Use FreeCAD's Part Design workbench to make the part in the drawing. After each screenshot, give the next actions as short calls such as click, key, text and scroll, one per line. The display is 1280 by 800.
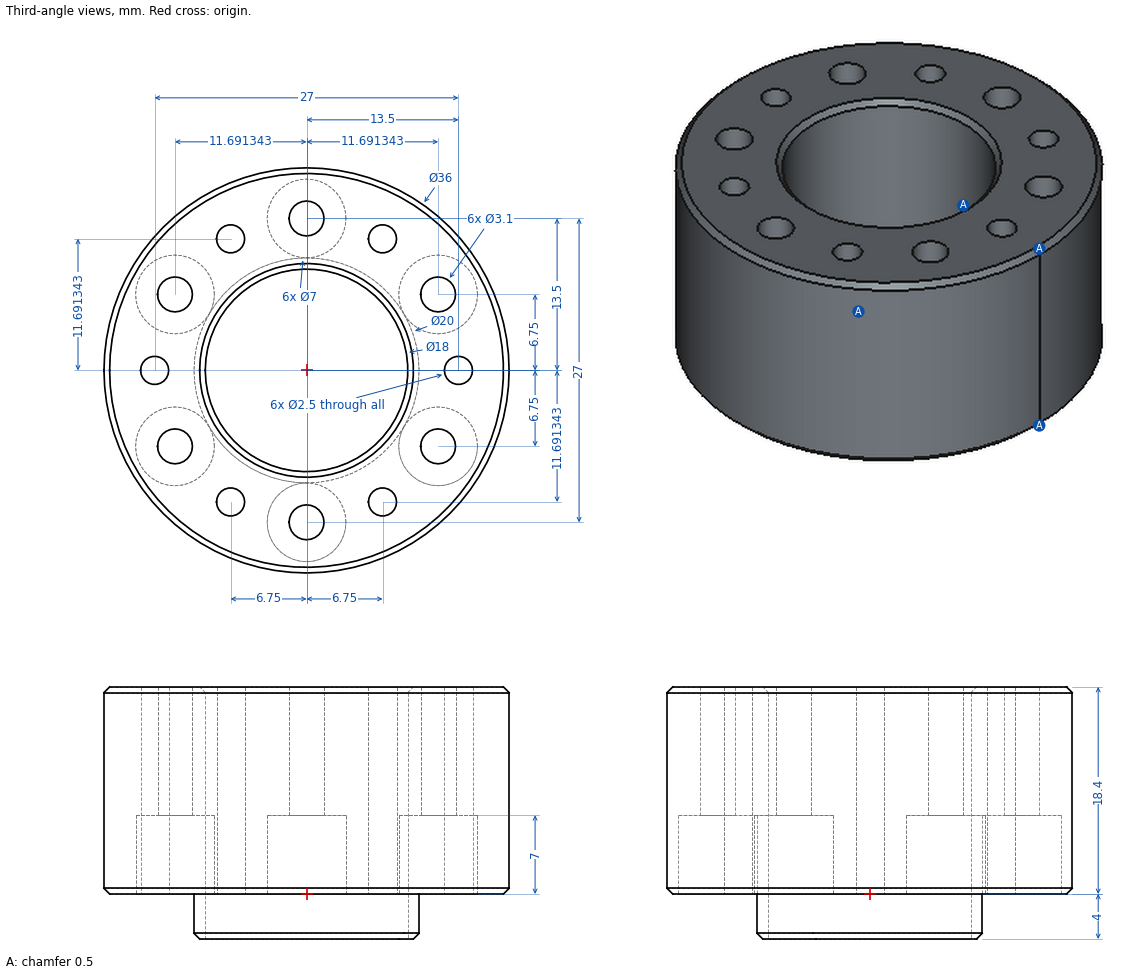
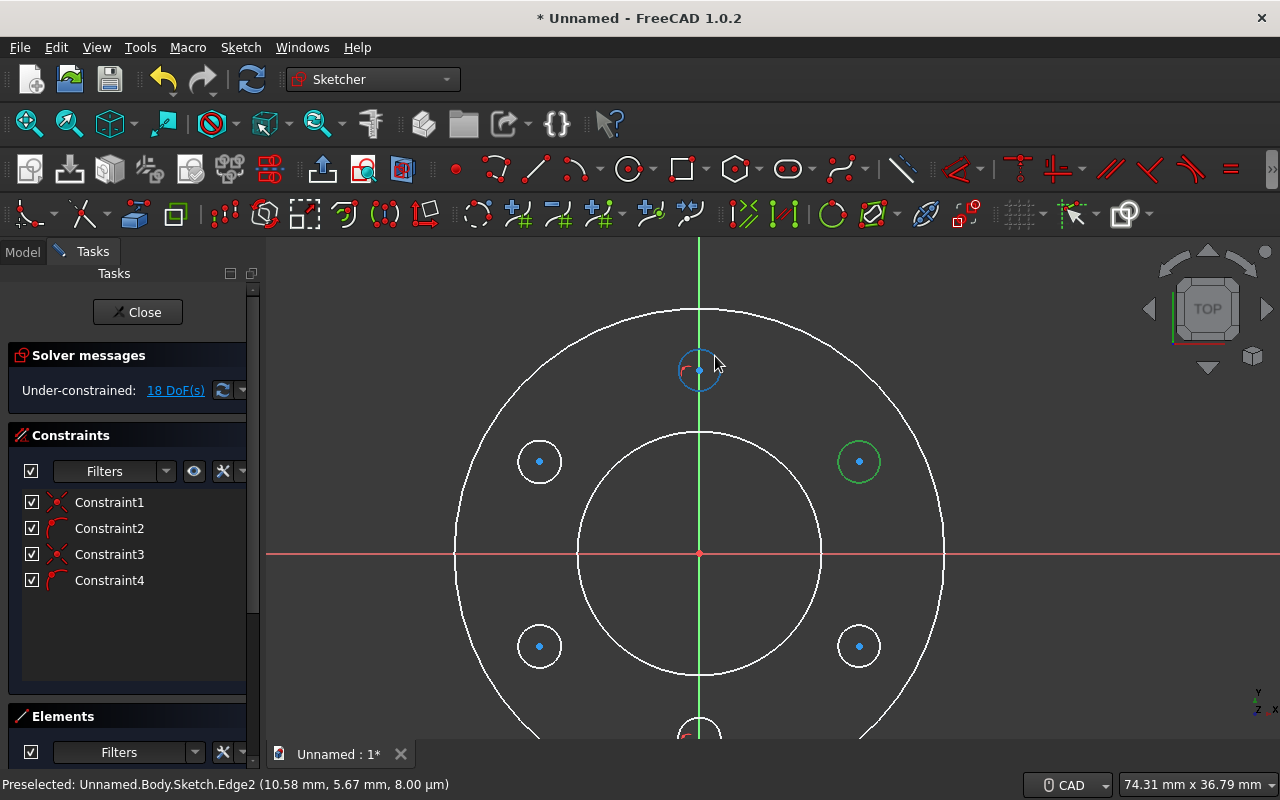
click(714, 355)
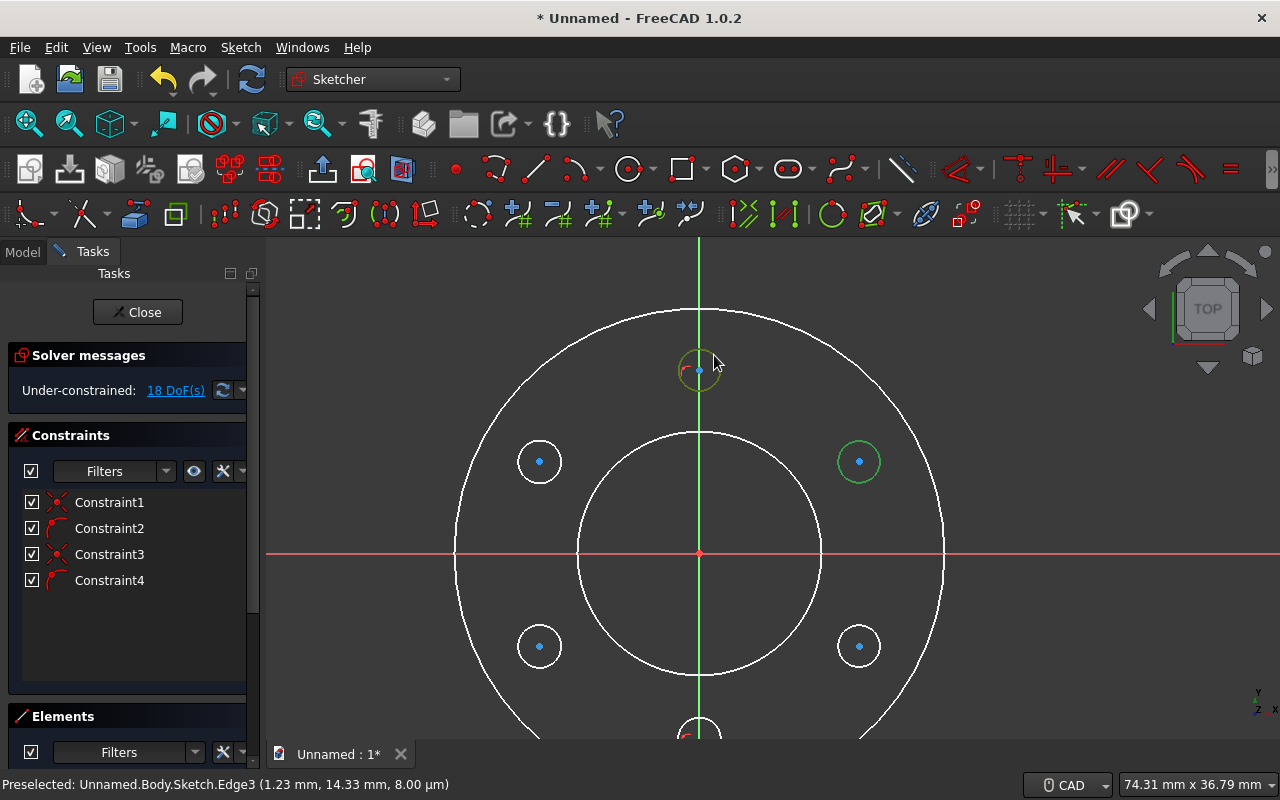
click(555, 447)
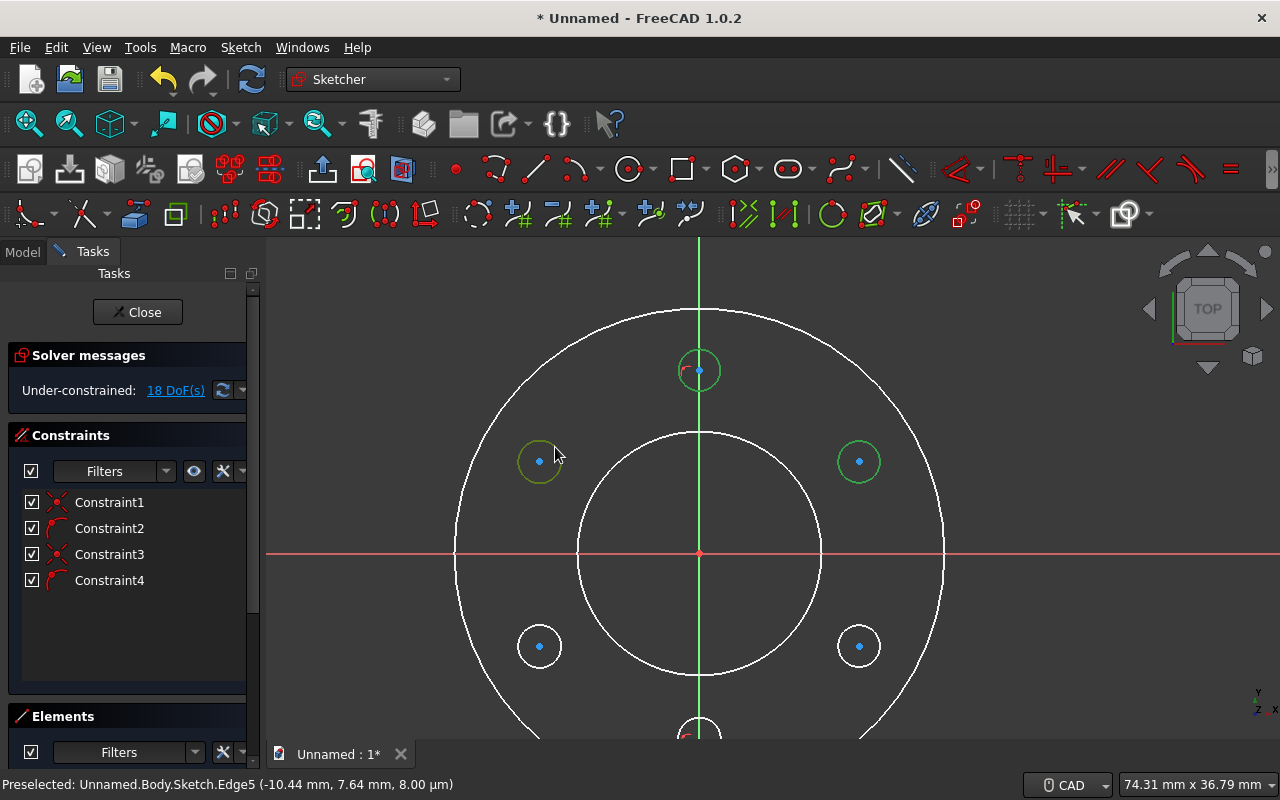
click(874, 631)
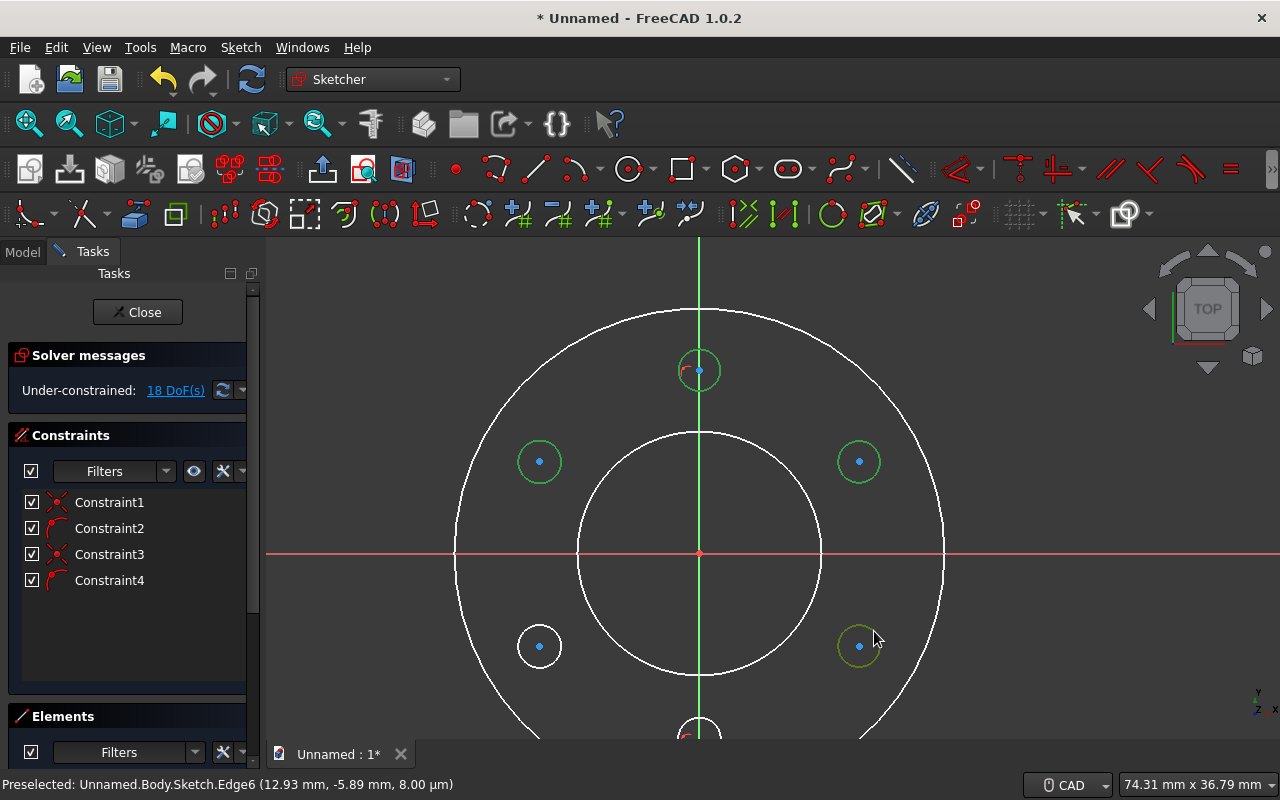
scroll(715, 355, down, 2)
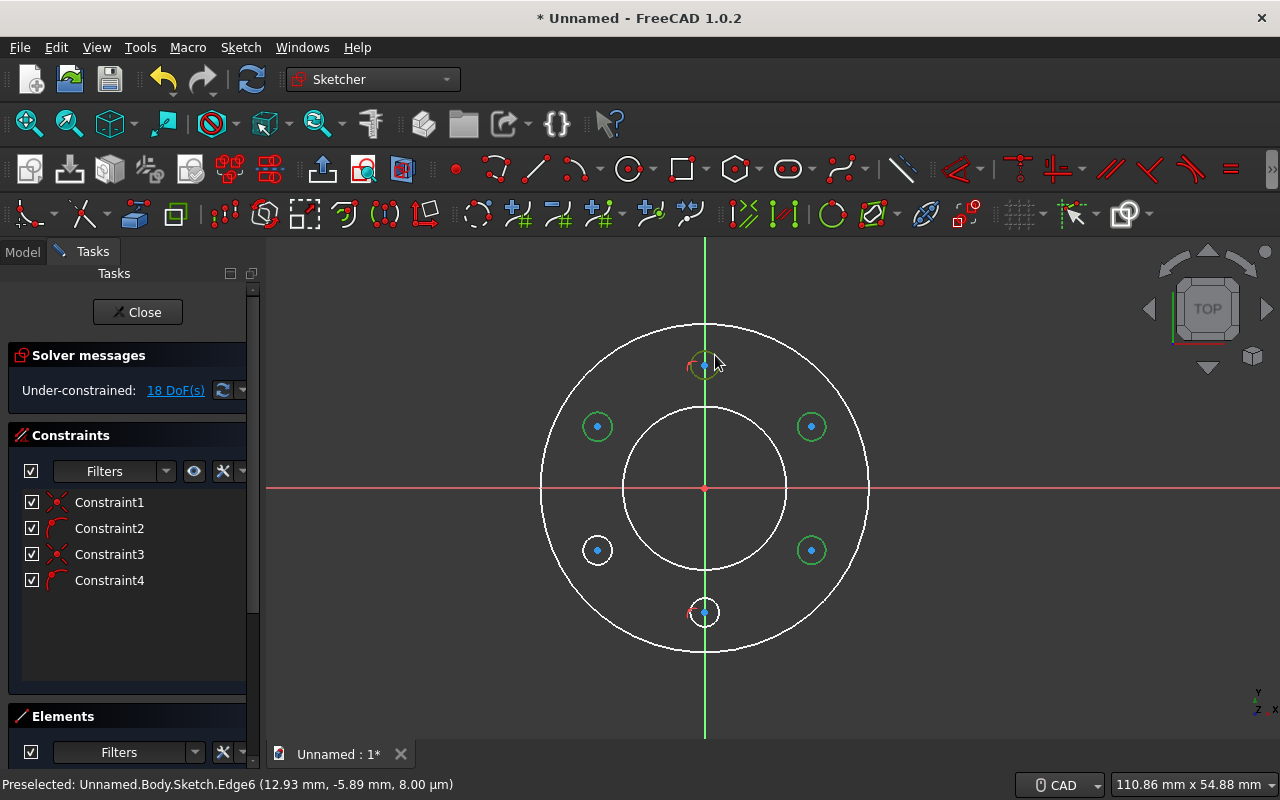
scroll(715, 602, up, 2)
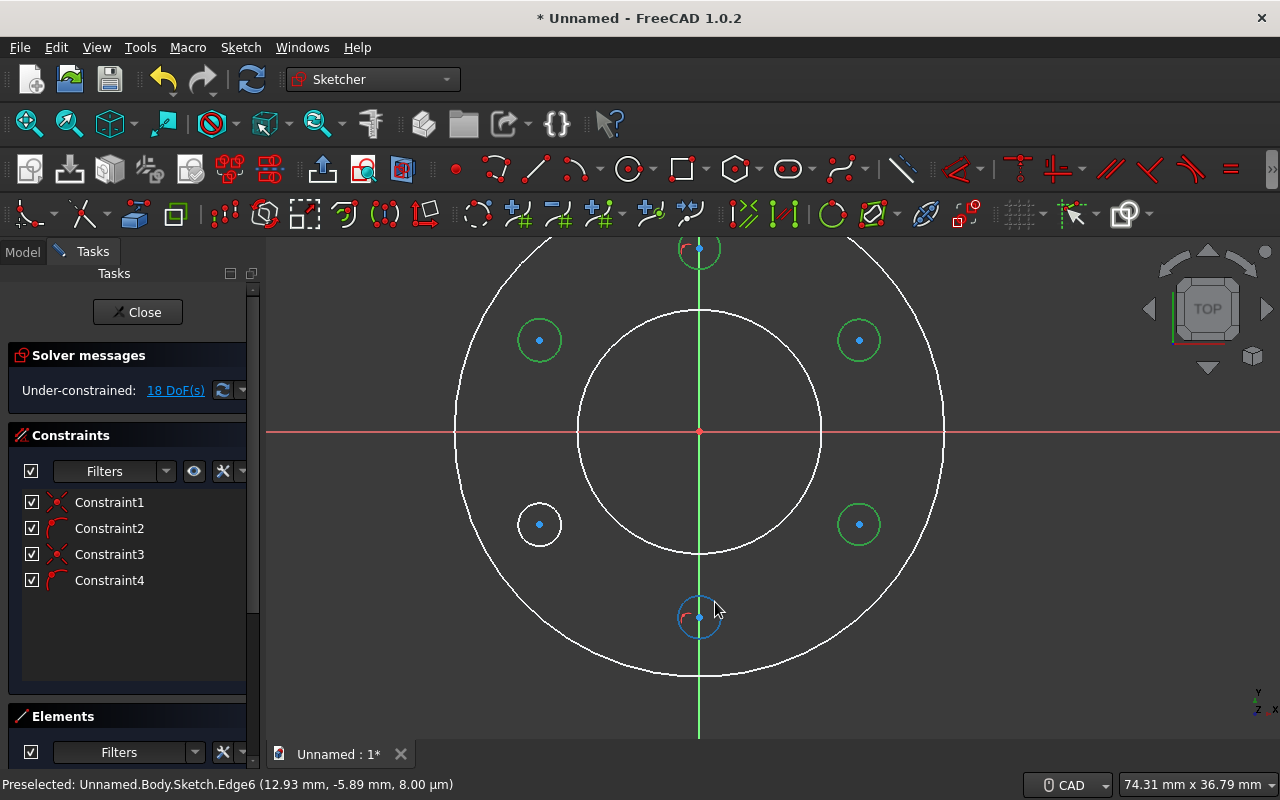
click(715, 602)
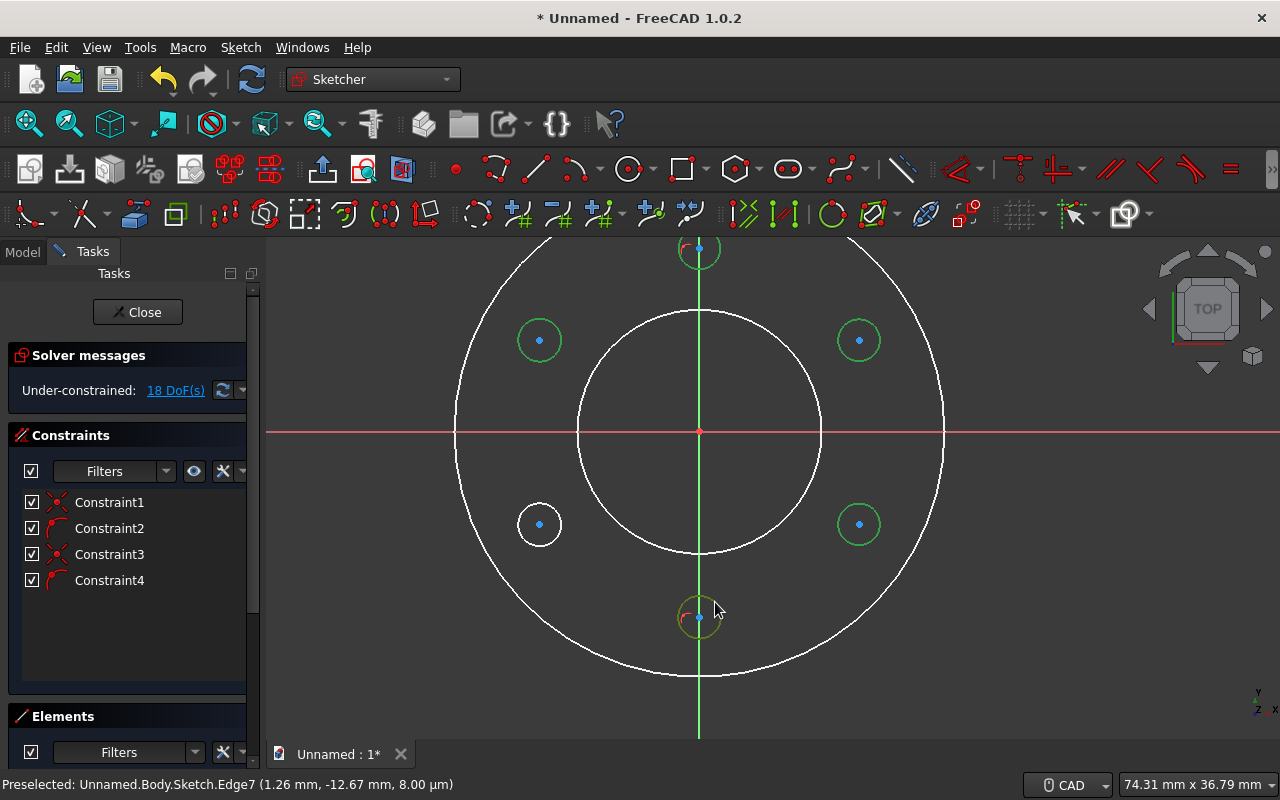
click(555, 510)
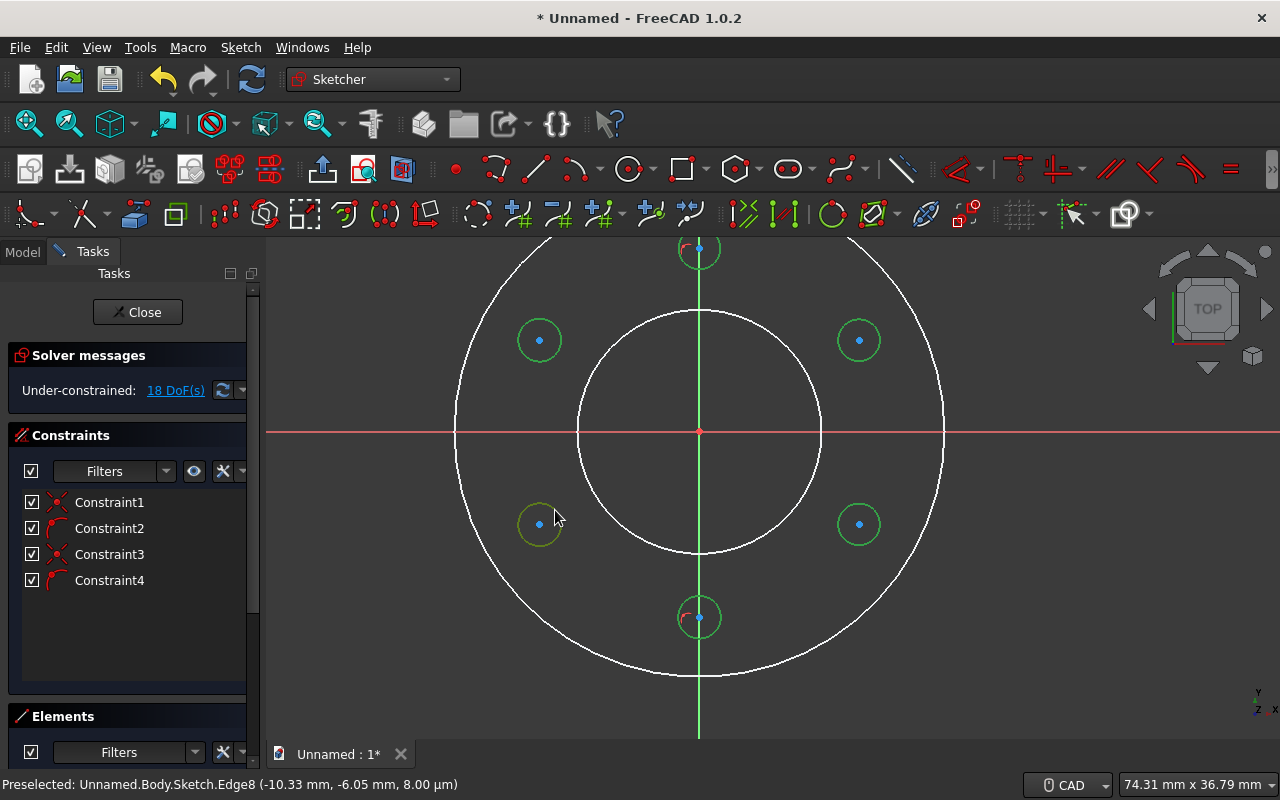
key(e)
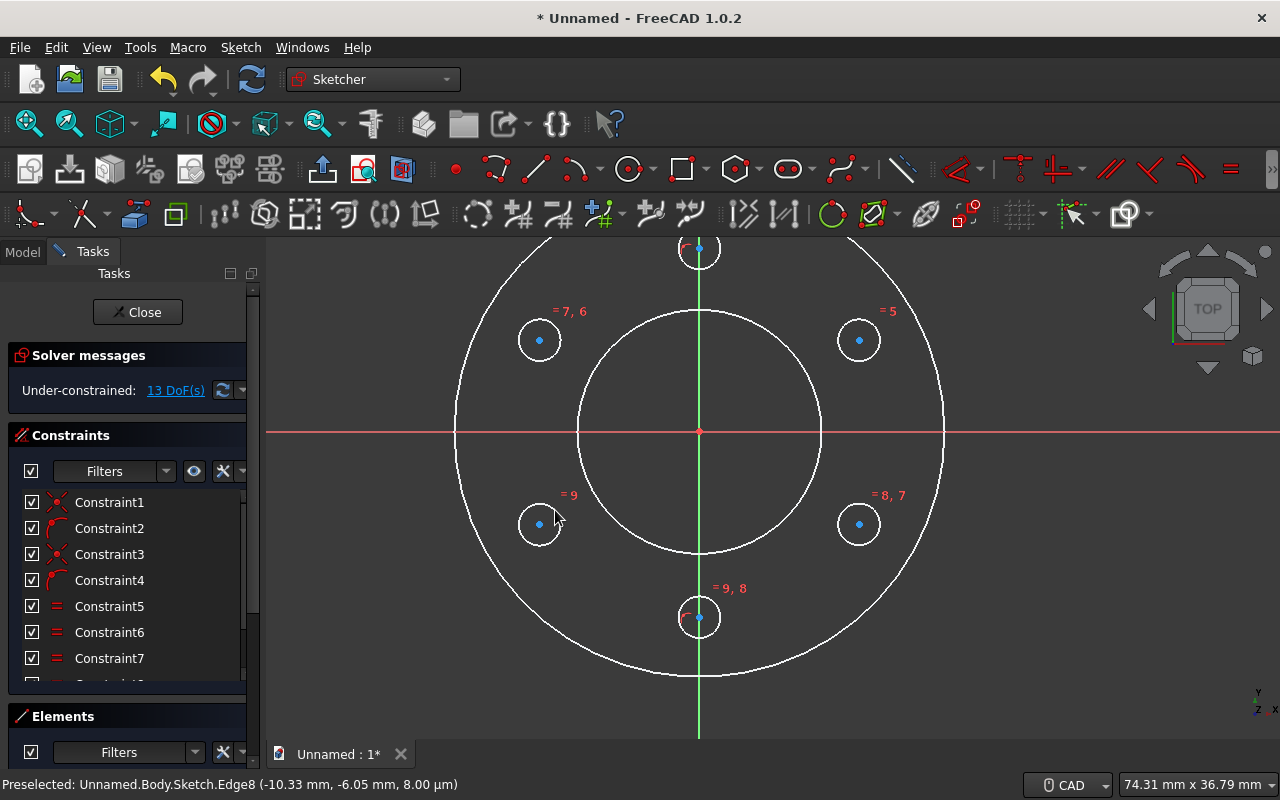
click(527, 606)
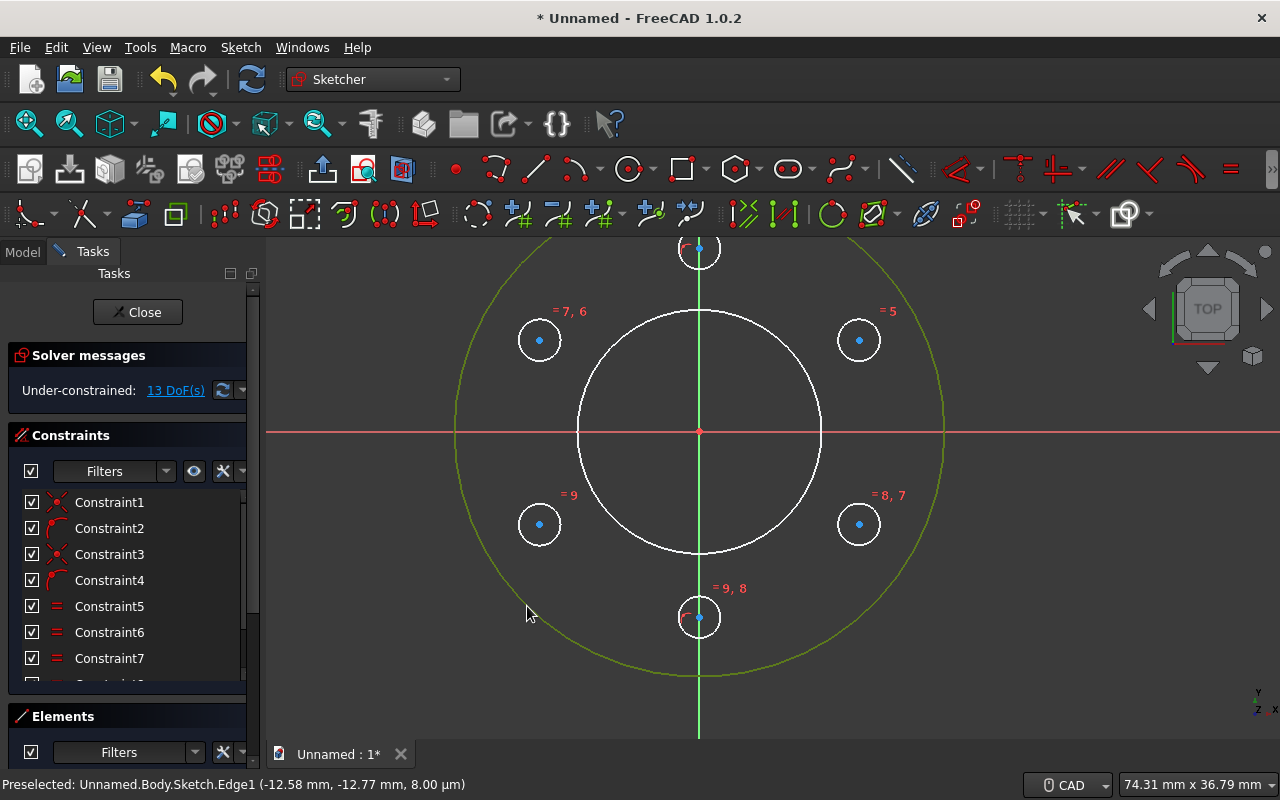
key(k)
key(o)